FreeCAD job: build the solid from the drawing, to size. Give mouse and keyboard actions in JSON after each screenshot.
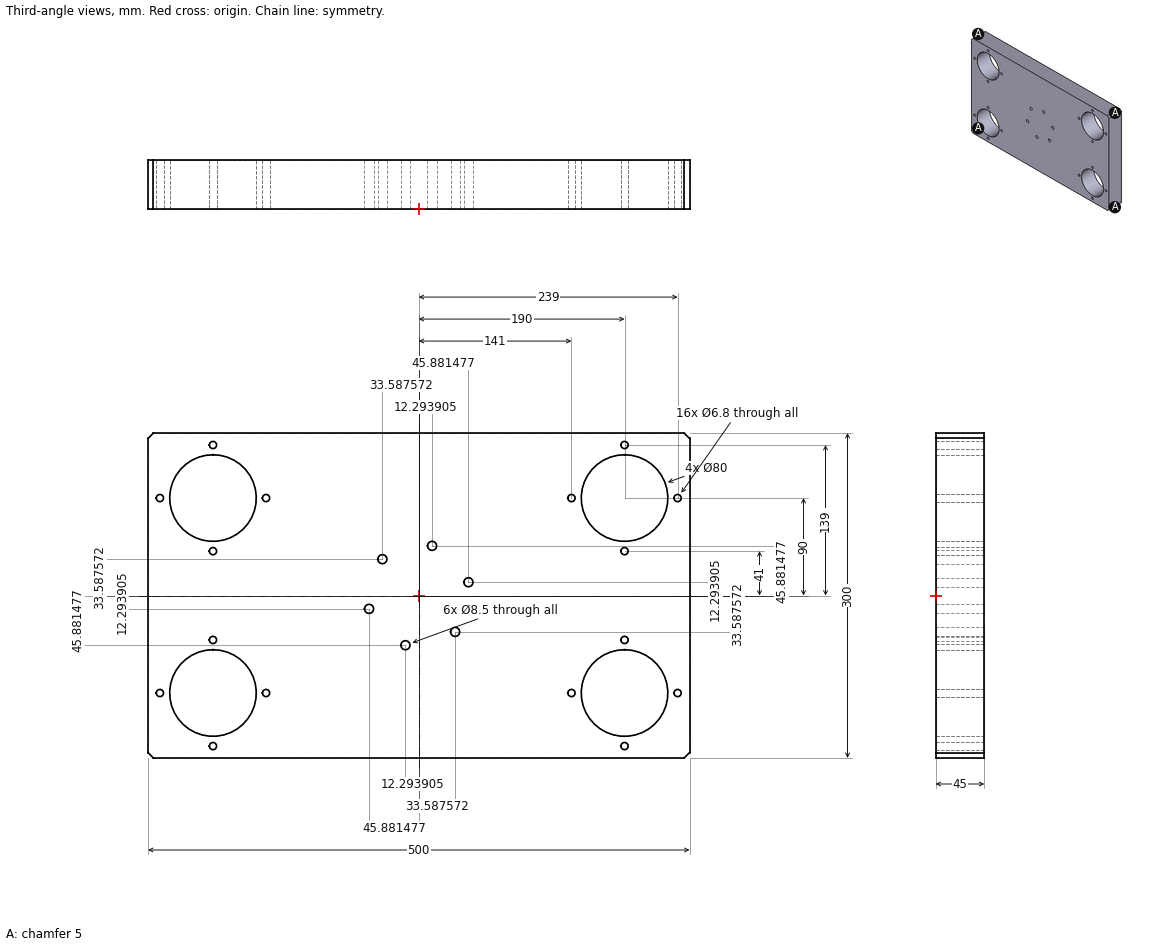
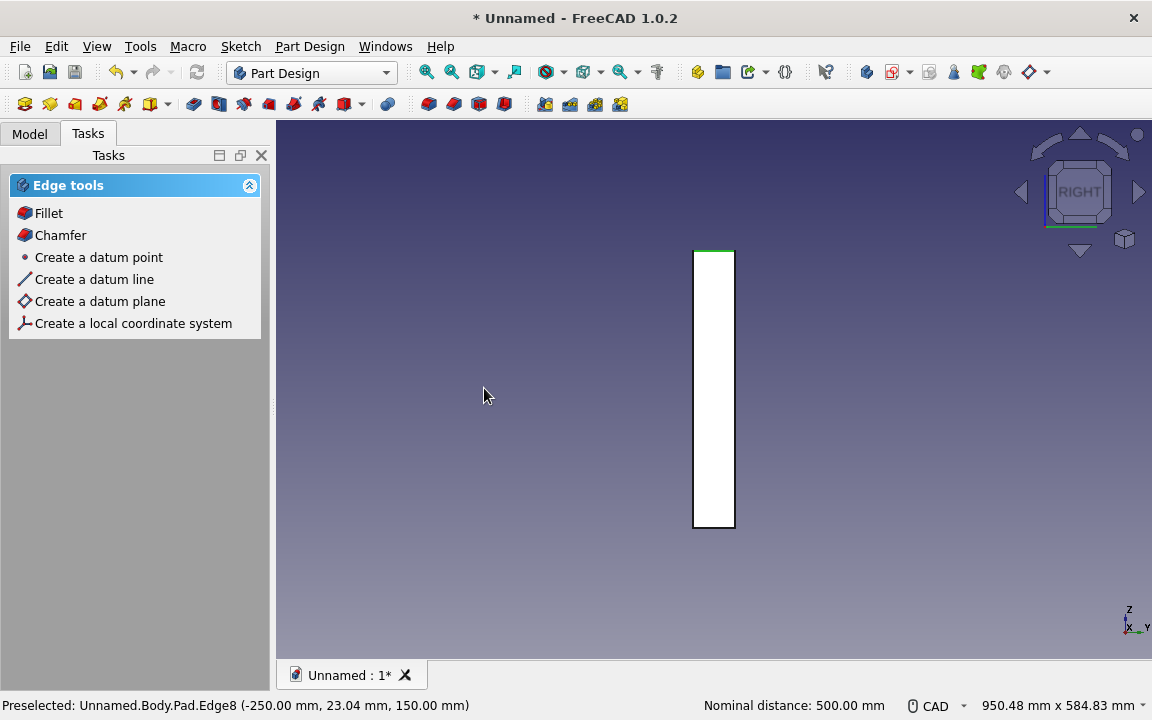
{"action": "left_click", "coordinate": [714, 527], "text": "ctrl"}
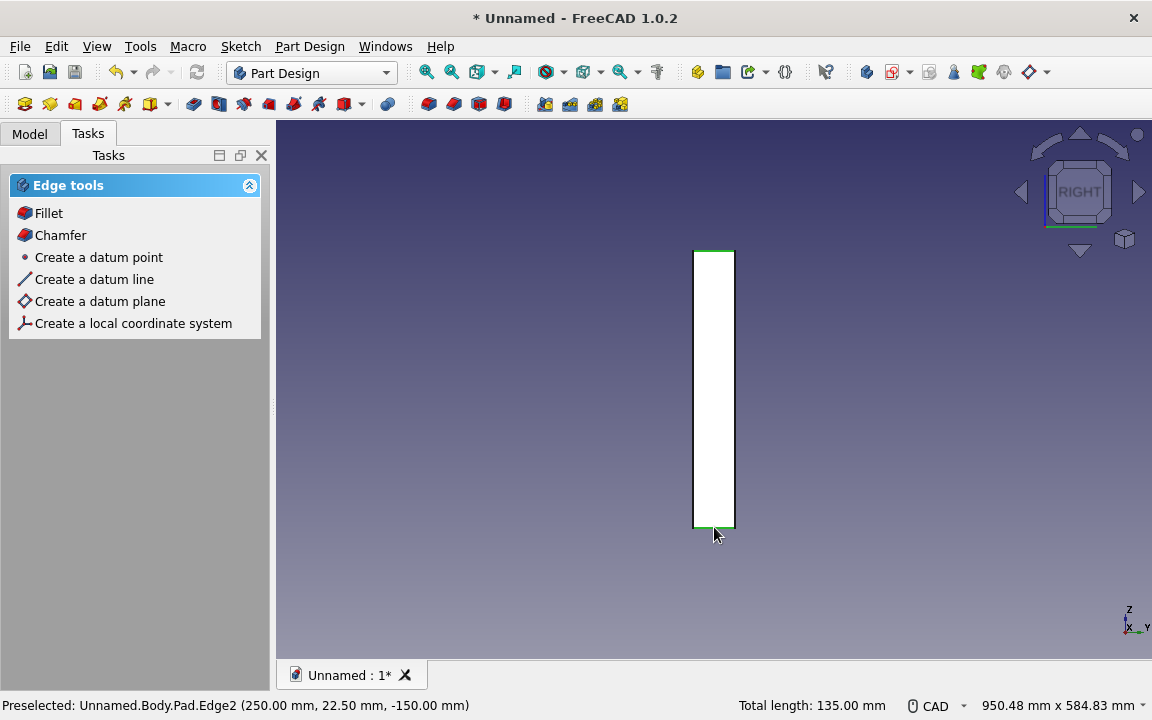
{"action": "key", "text": "5"}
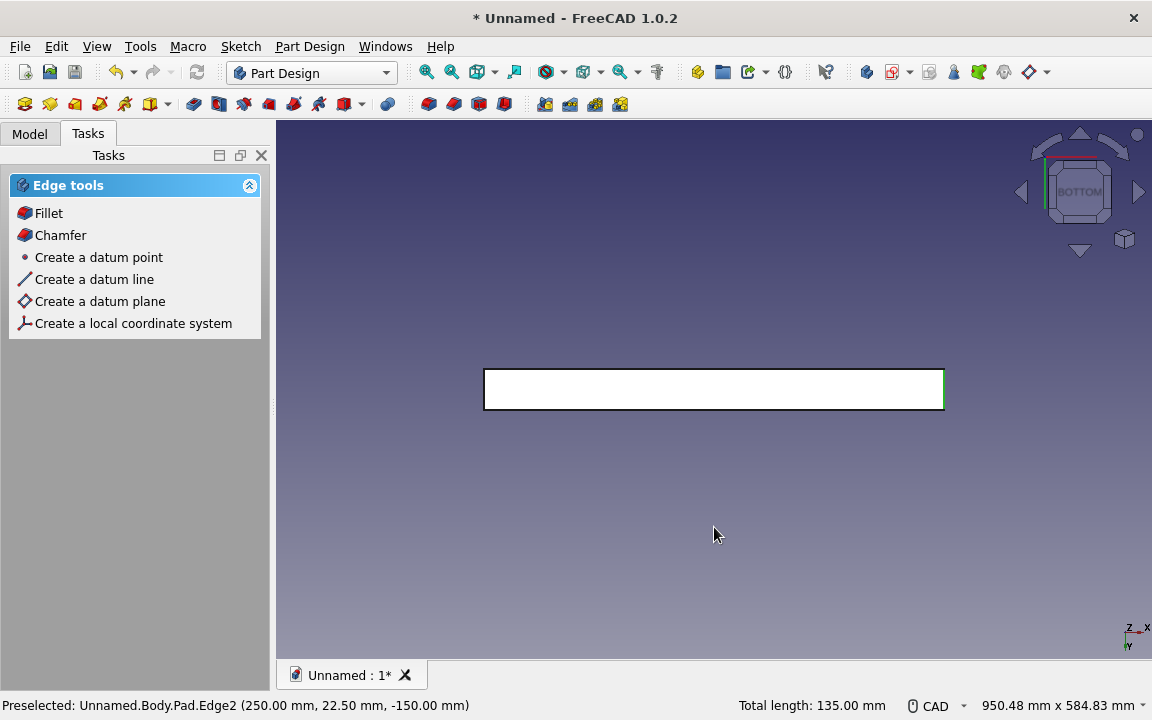
{"action": "left_click", "coordinate": [484, 388], "text": "ctrl"}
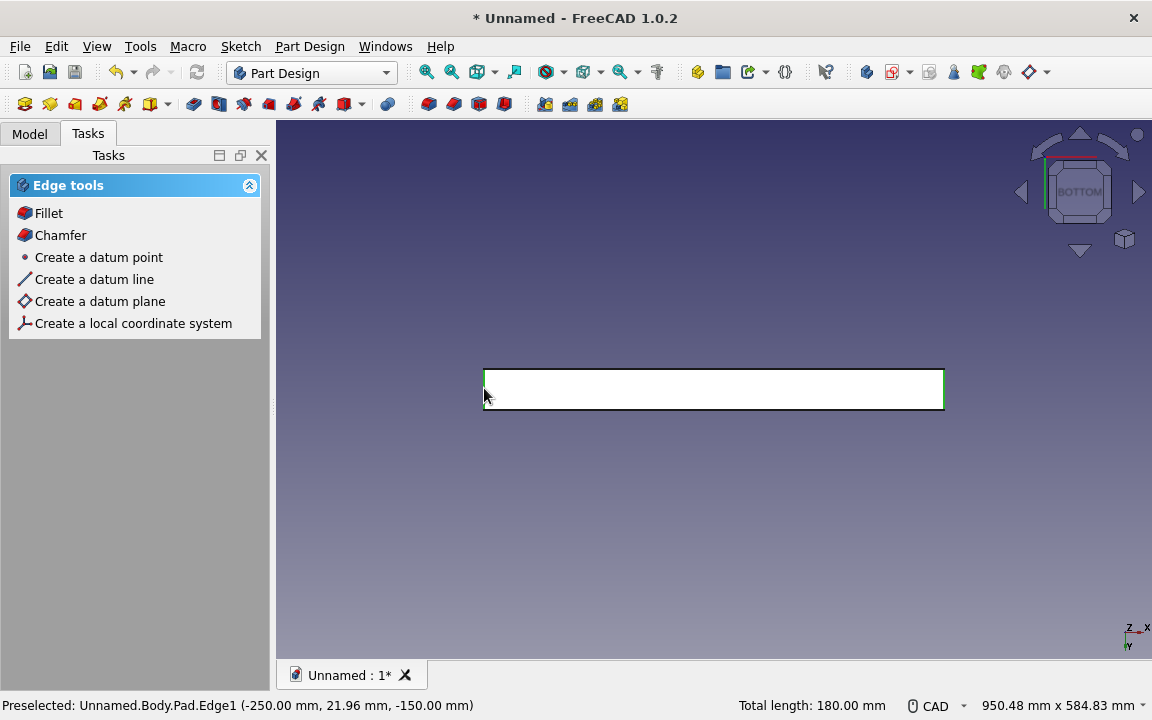
{"action": "left_click", "coordinate": [454, 104]}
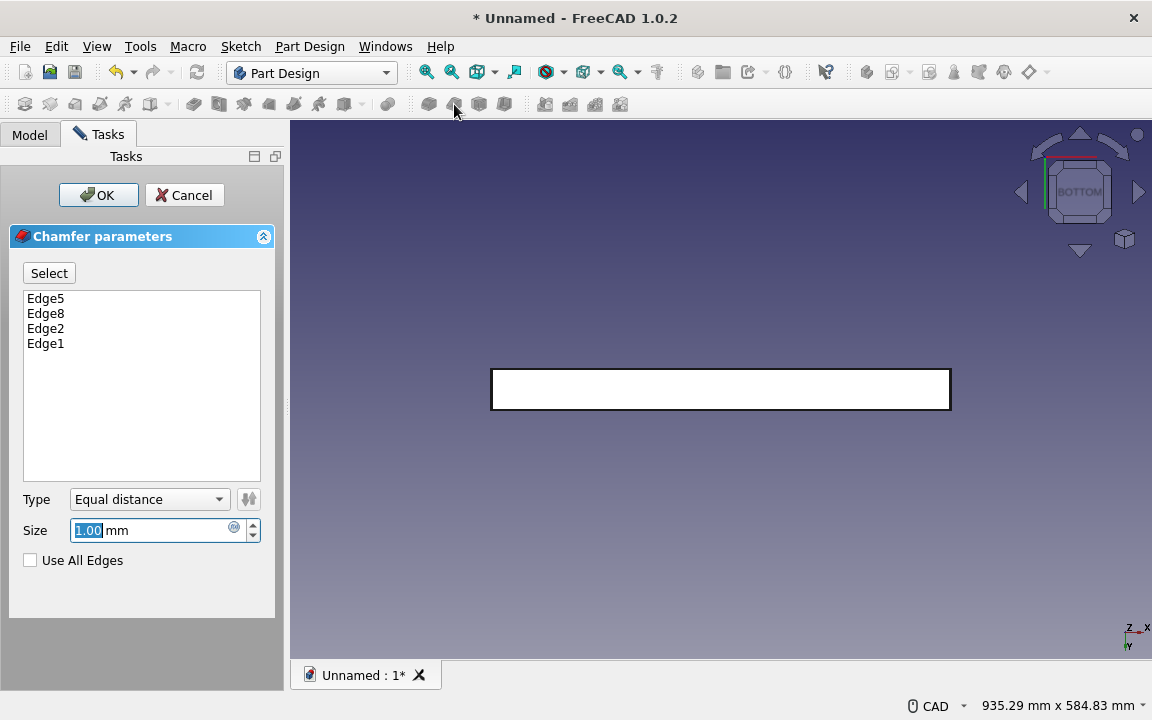
{"action": "type", "text": "5"}
{"action": "key", "text": "Tab"}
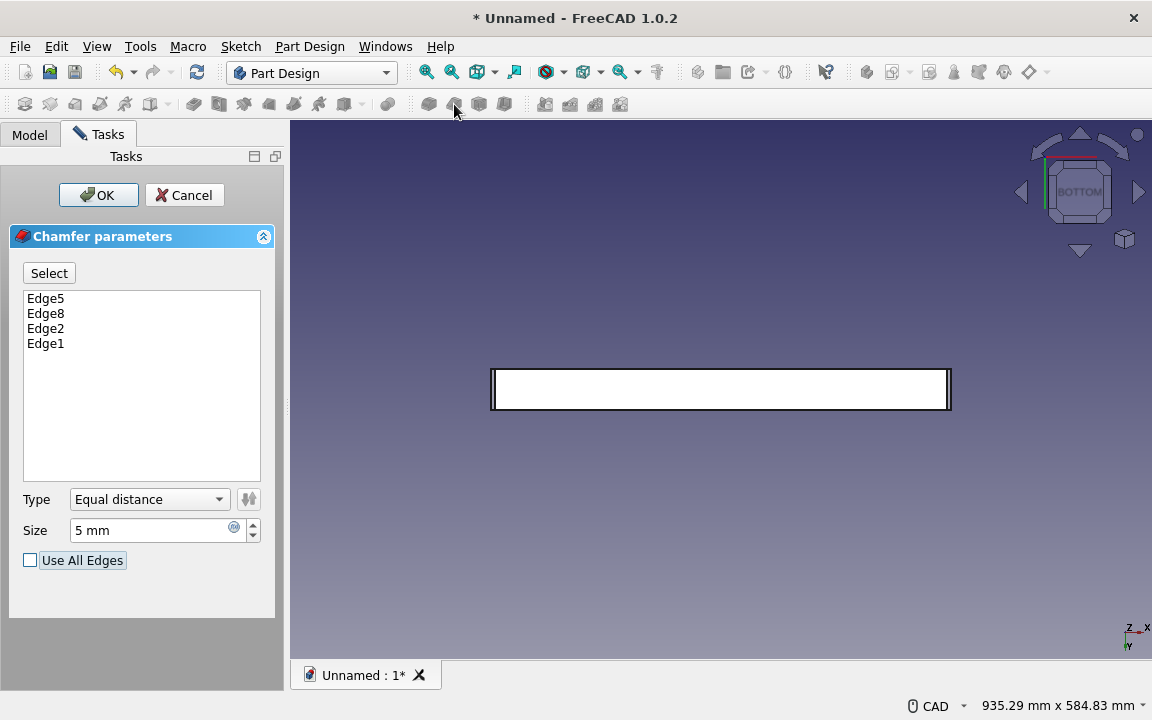
{"action": "left_click", "coordinate": [99, 195]}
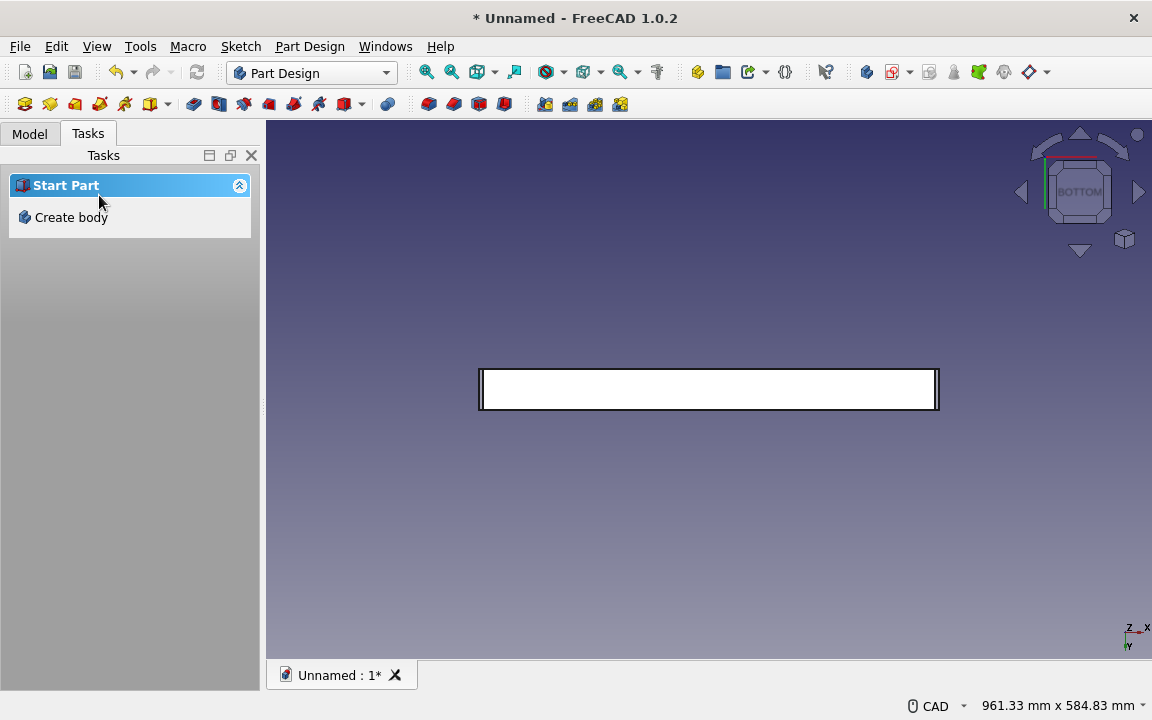
{"action": "key", "text": "4"}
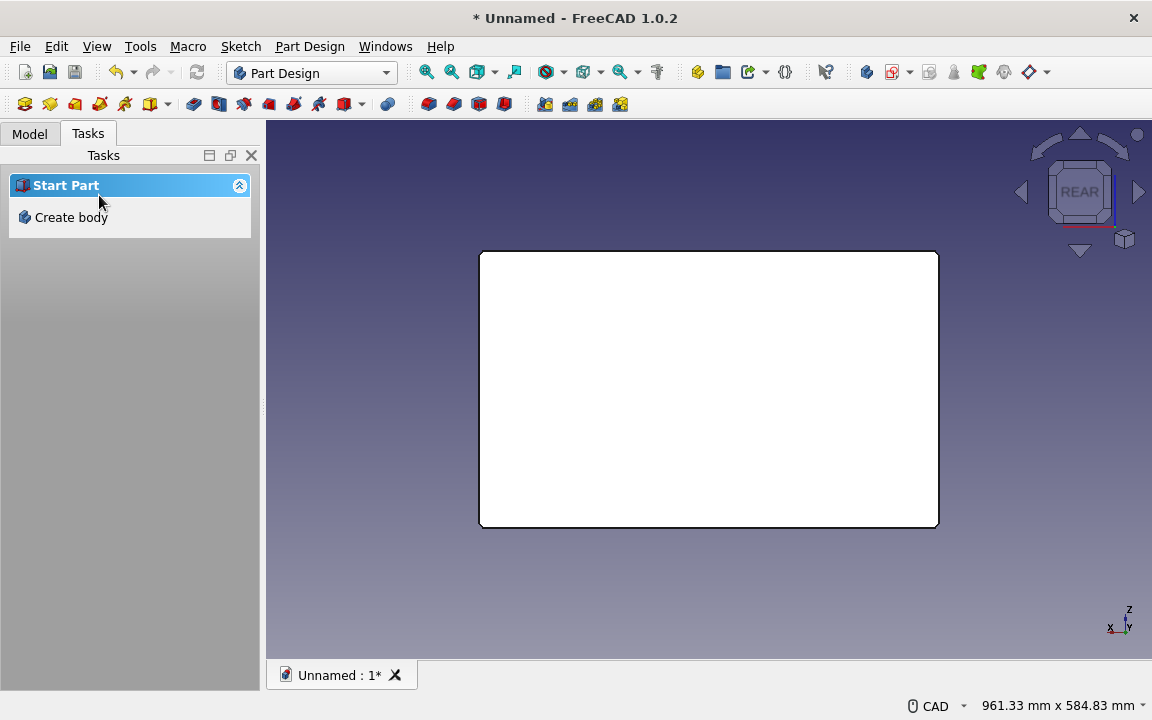
{"action": "left_click", "coordinate": [643, 389]}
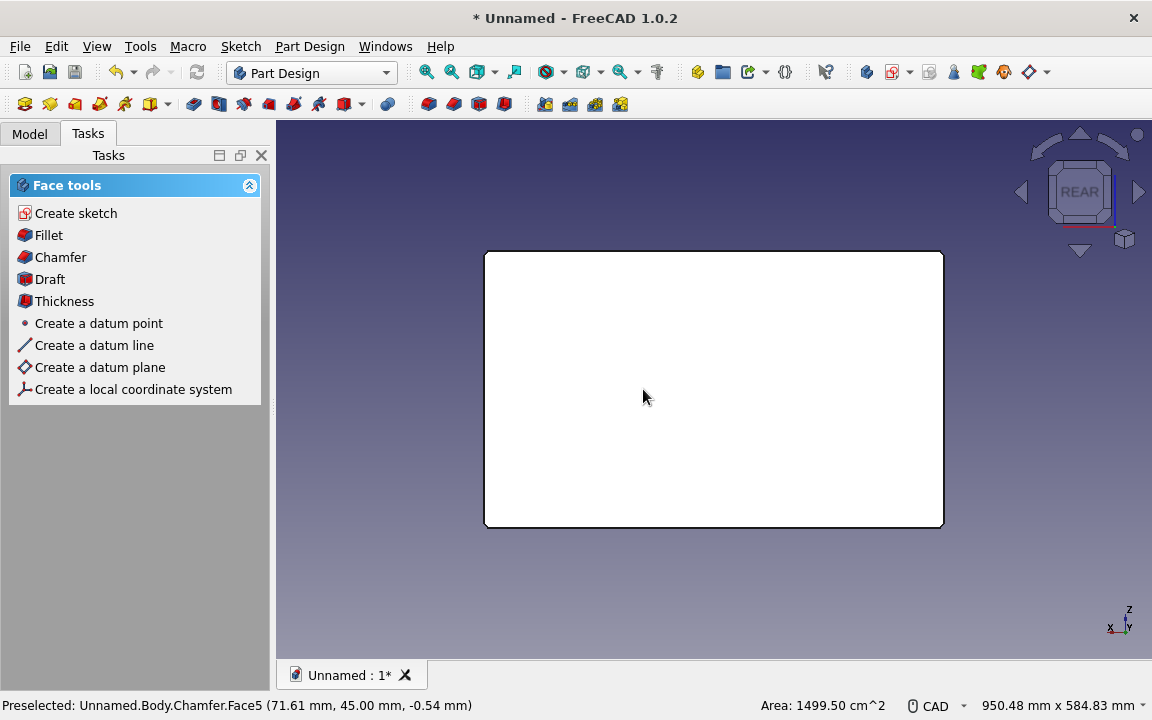
{"action": "left_click", "coordinate": [892, 72]}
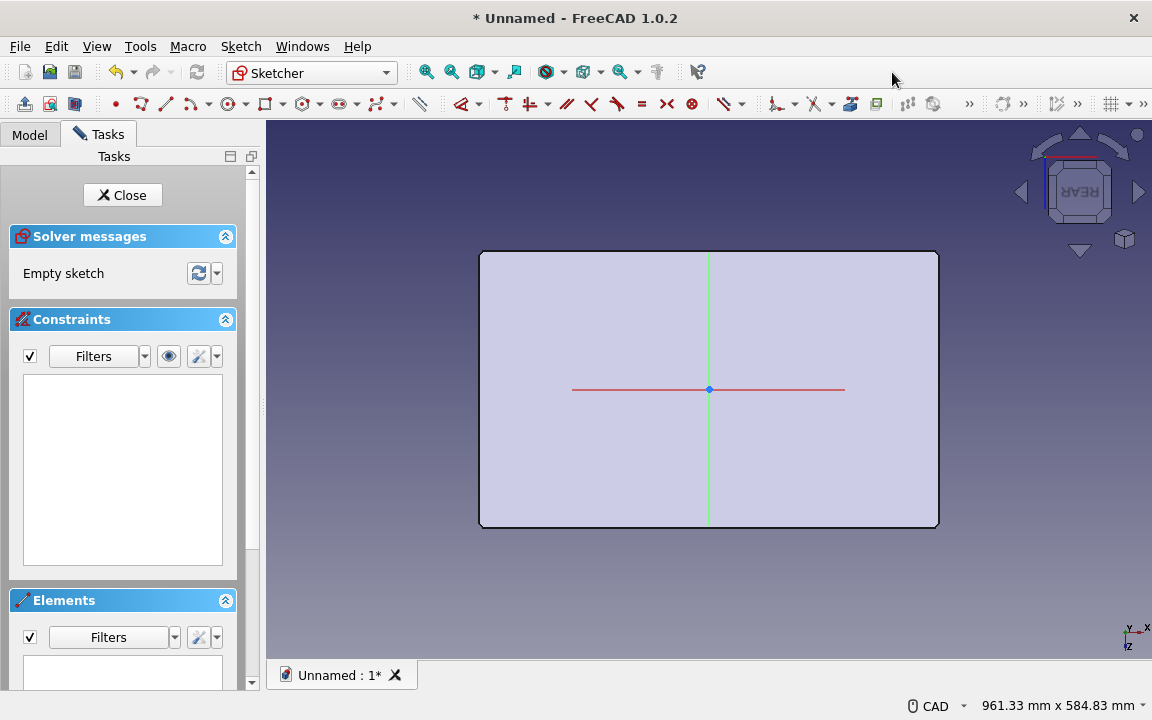
{"action": "left_click", "coordinate": [228, 104]}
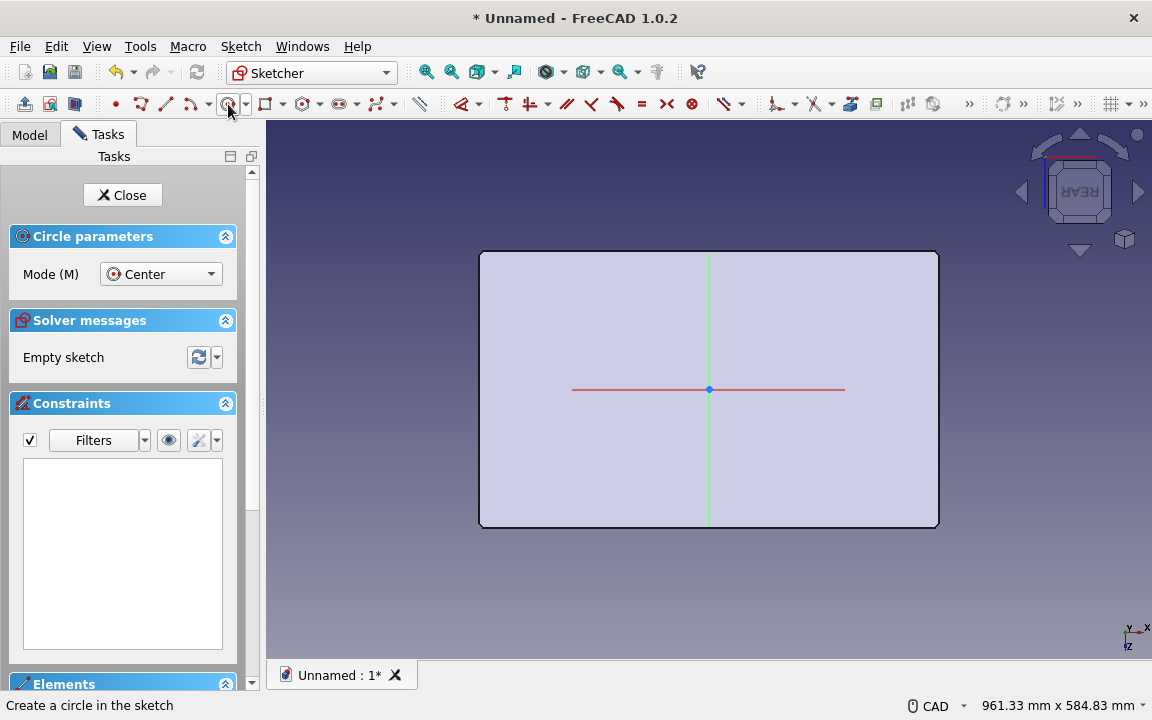
{"action": "left_click", "coordinate": [884, 472]}
{"action": "left_click", "coordinate": [910, 446]}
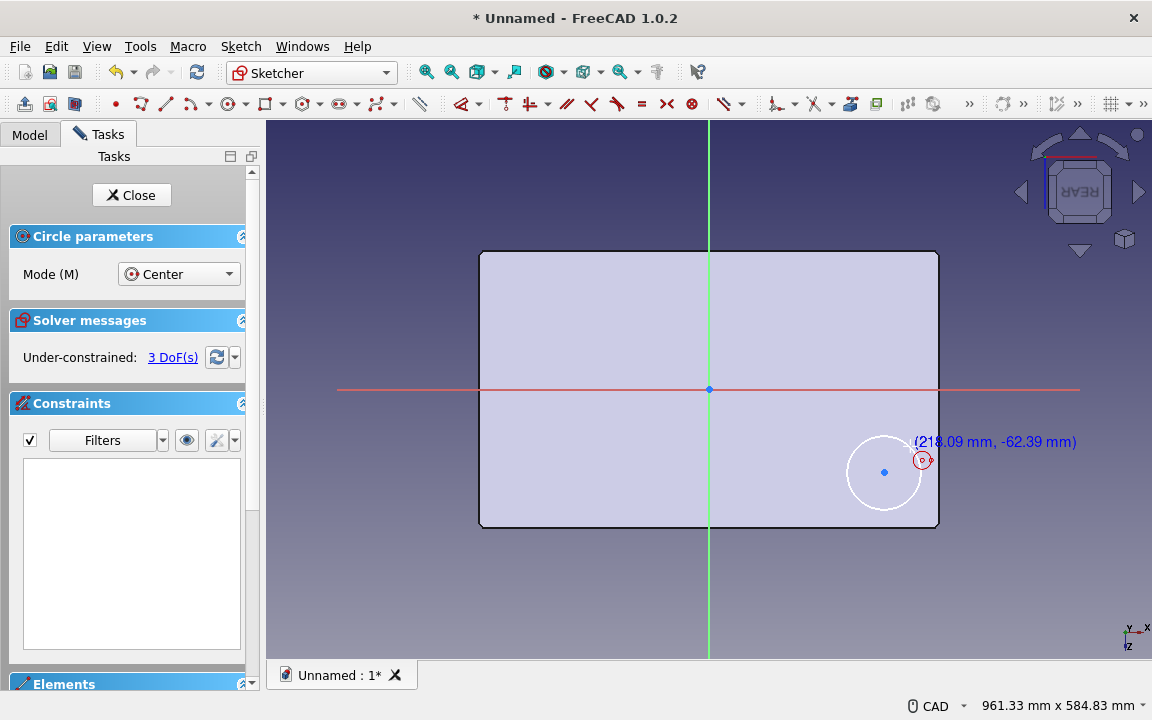
{"action": "left_click", "coordinate": [884, 307]}
{"action": "left_click", "coordinate": [910, 280]}